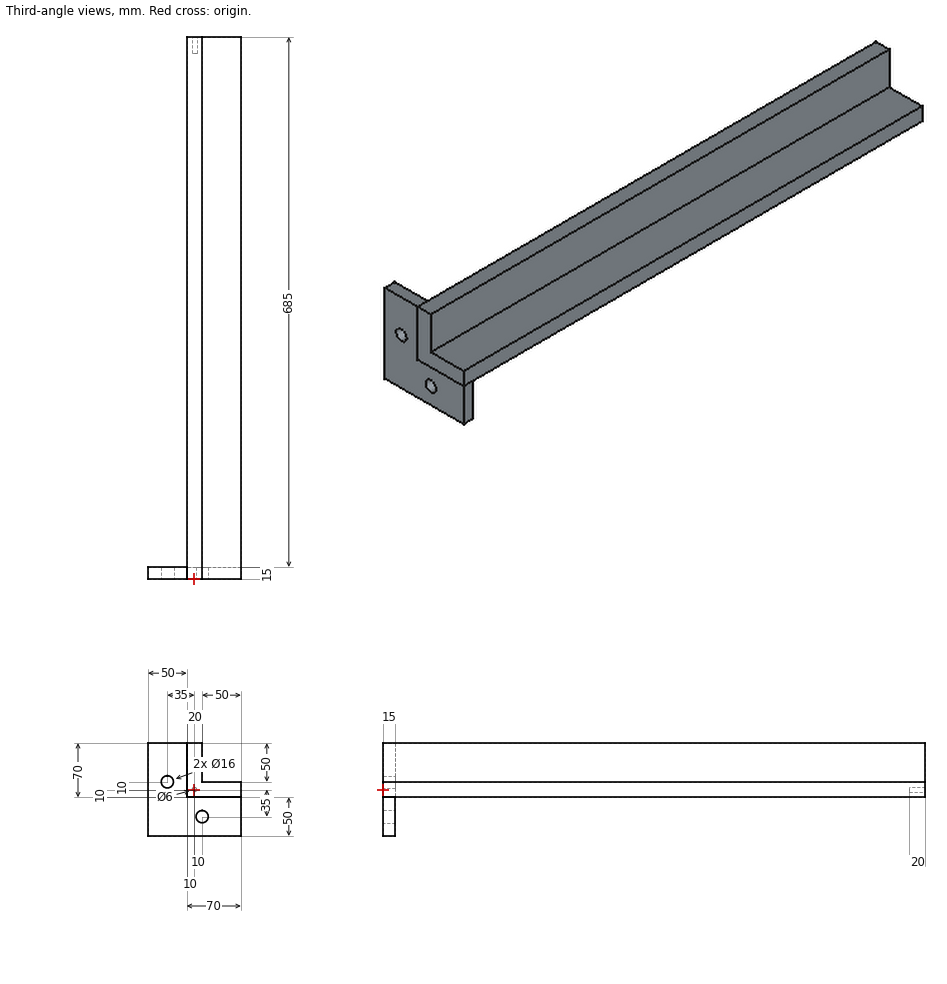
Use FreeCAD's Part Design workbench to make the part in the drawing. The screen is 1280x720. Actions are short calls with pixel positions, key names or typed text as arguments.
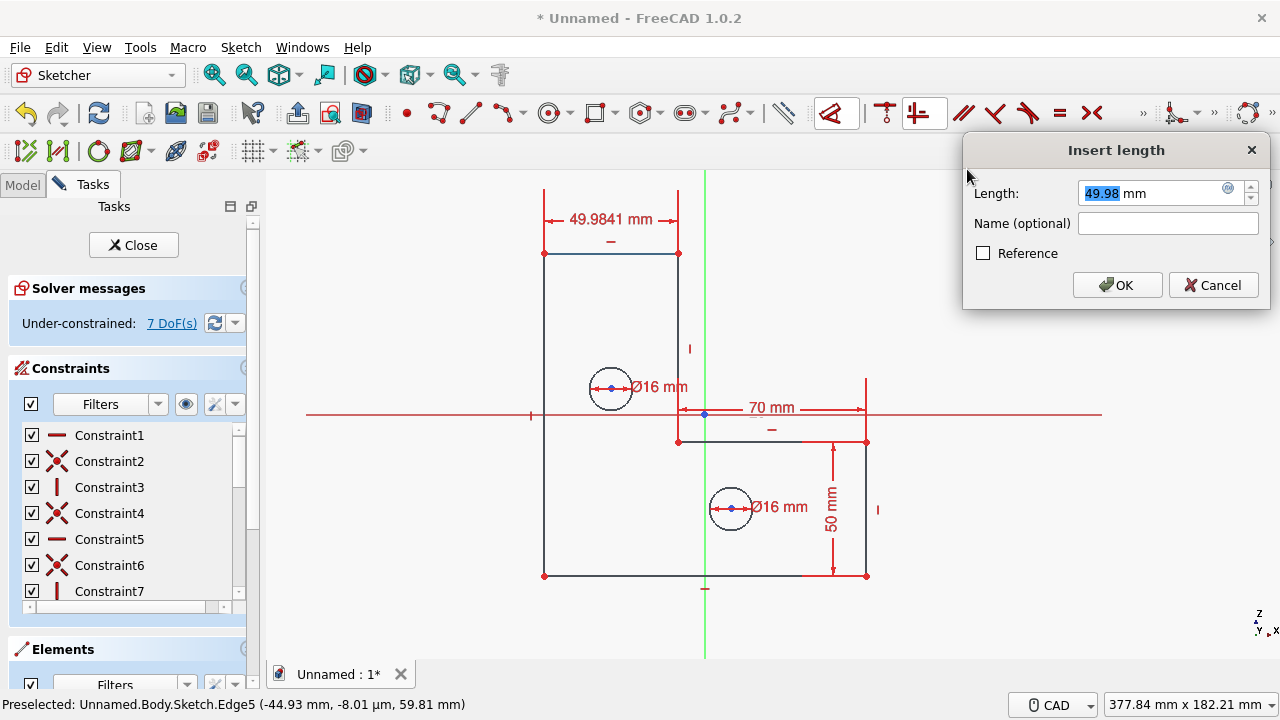
text(50)
key(Return)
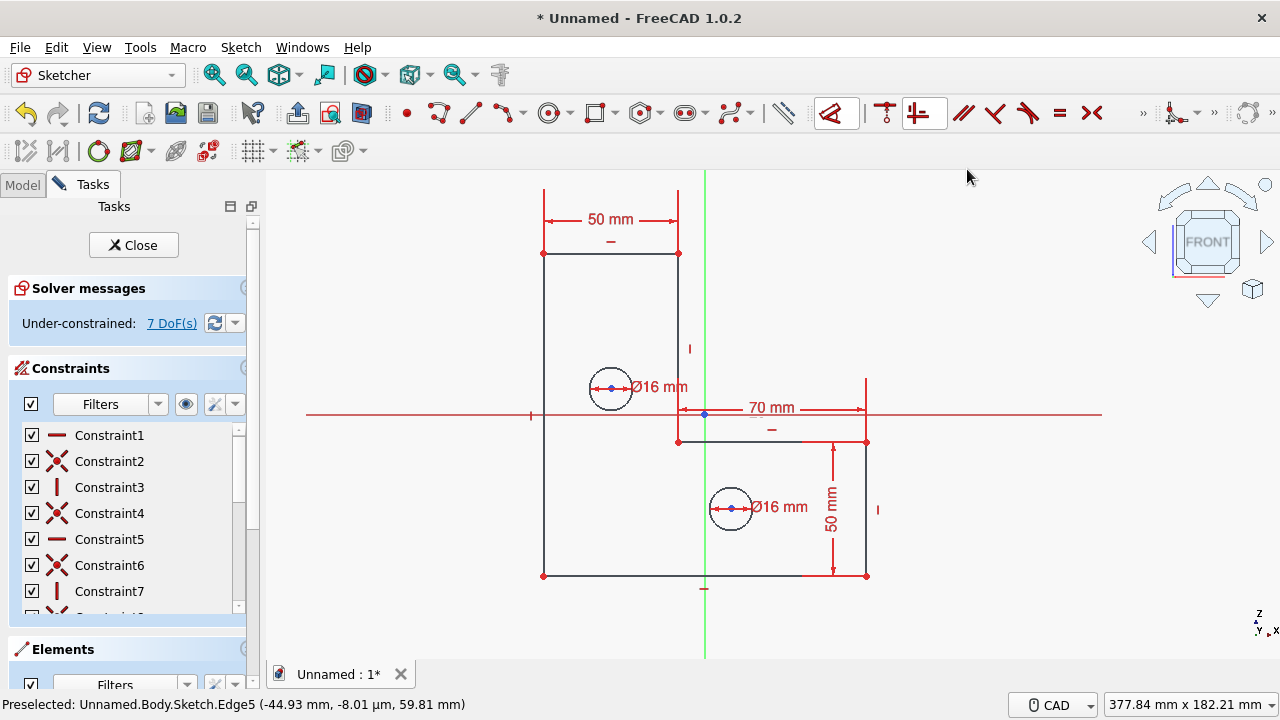
click(678, 310)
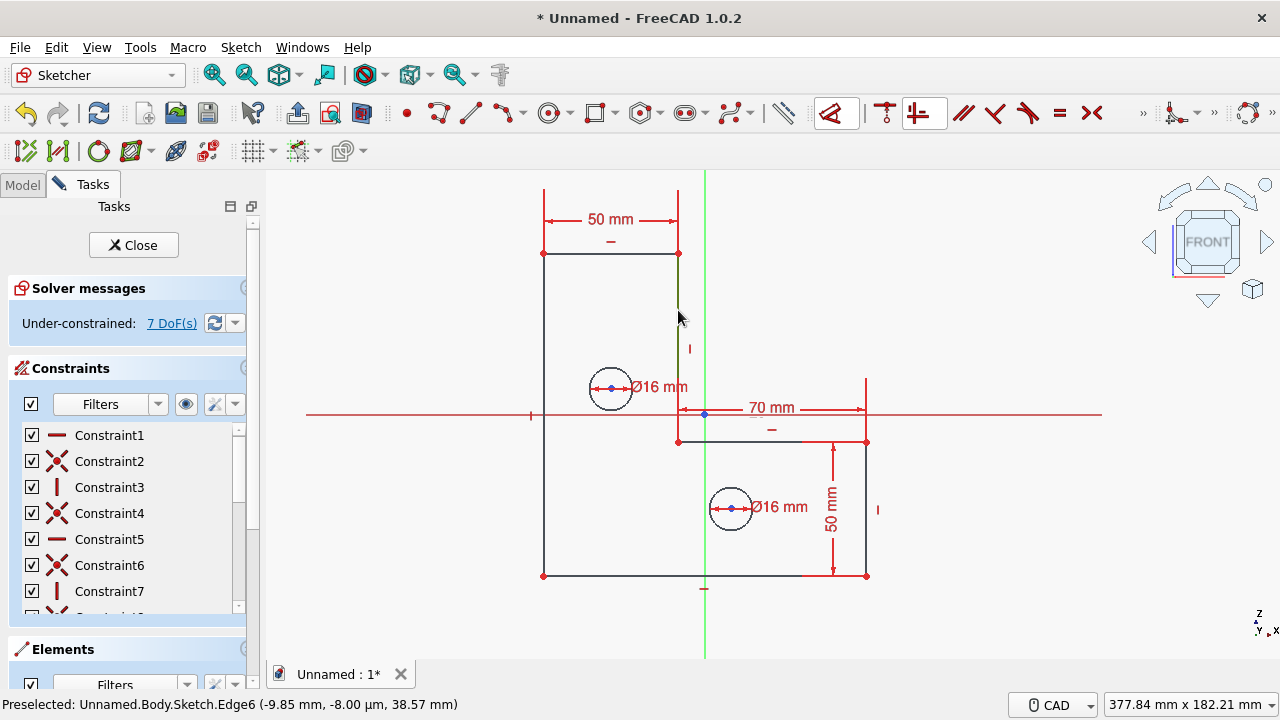
key(i)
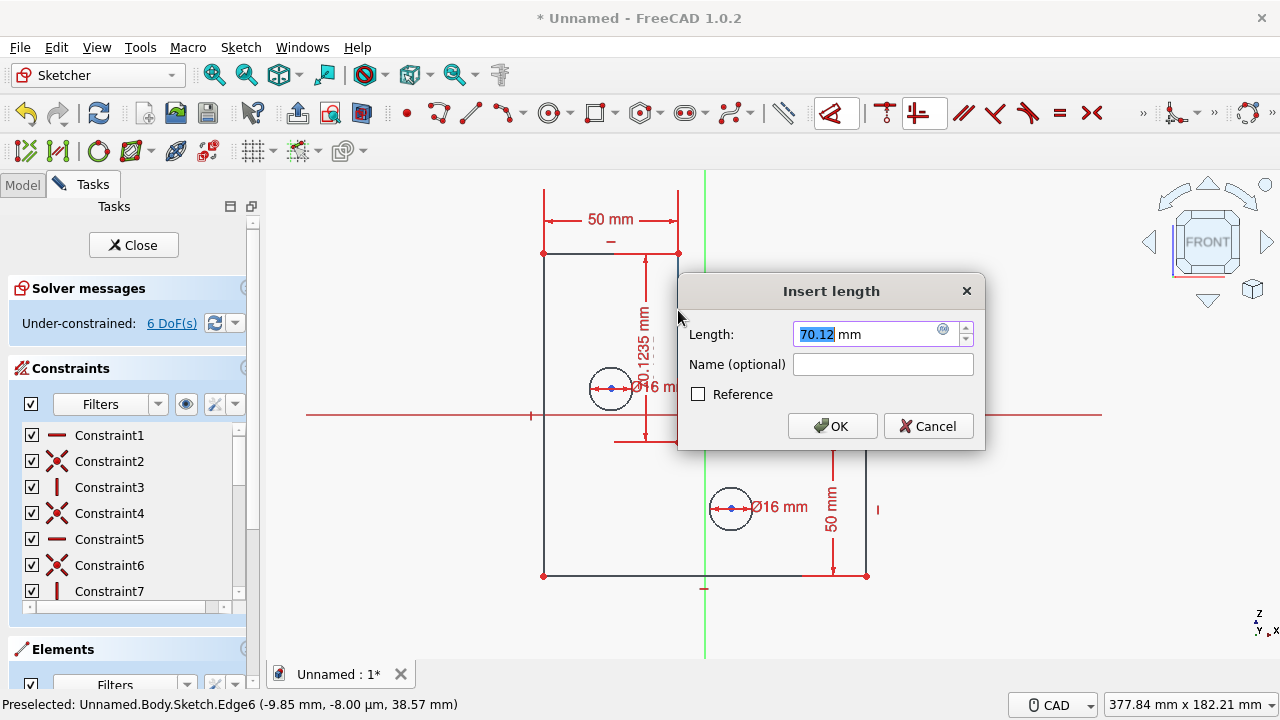
text(70)
key(Return)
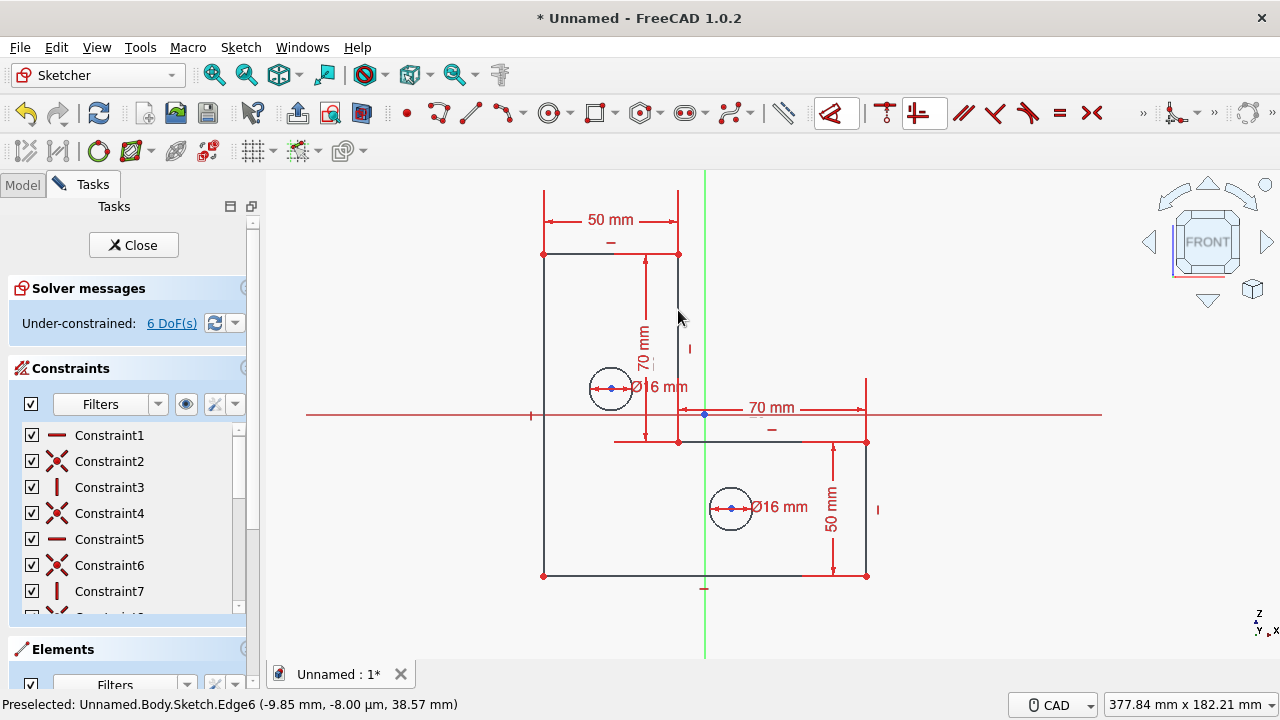
click(611, 389)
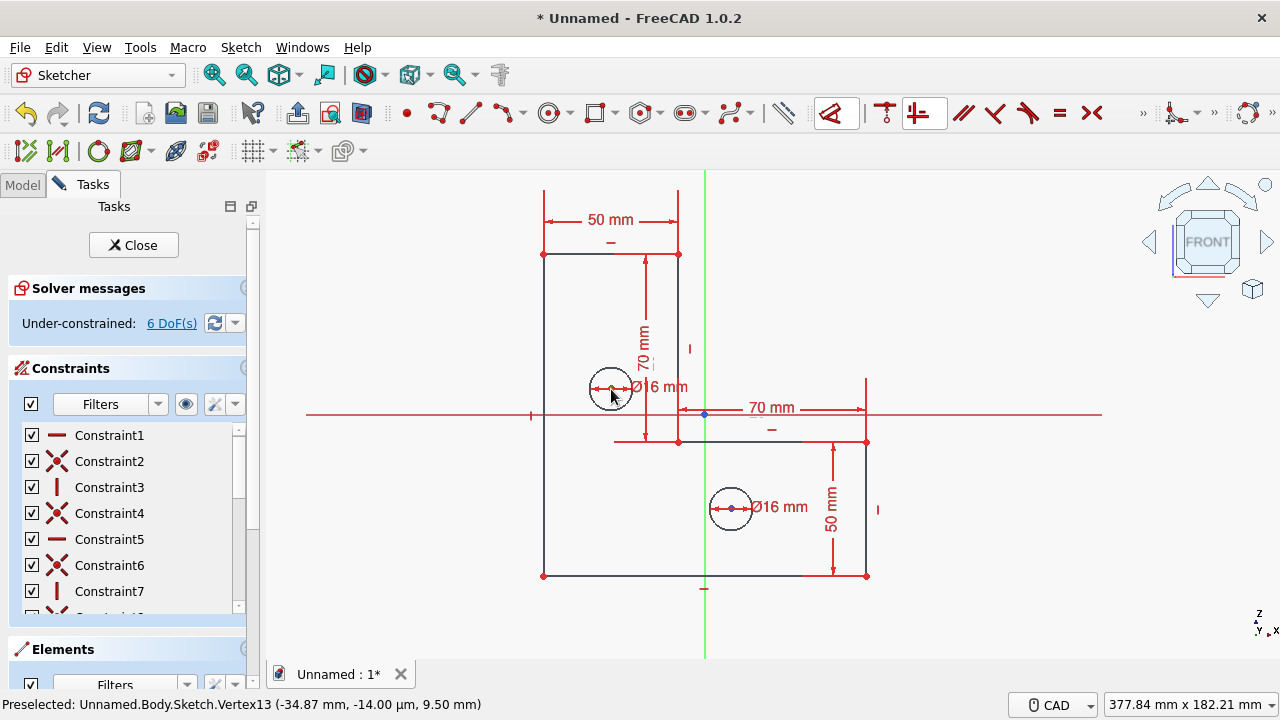
key(l)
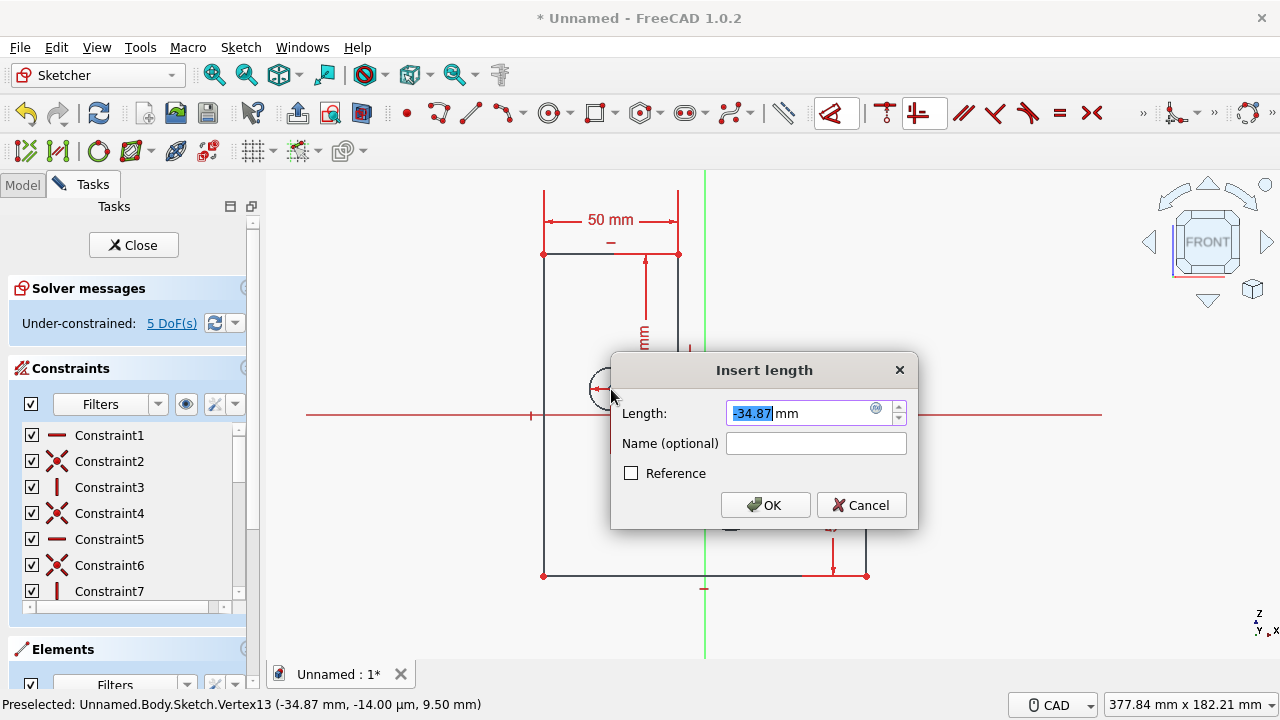
text(-35)
key(Return)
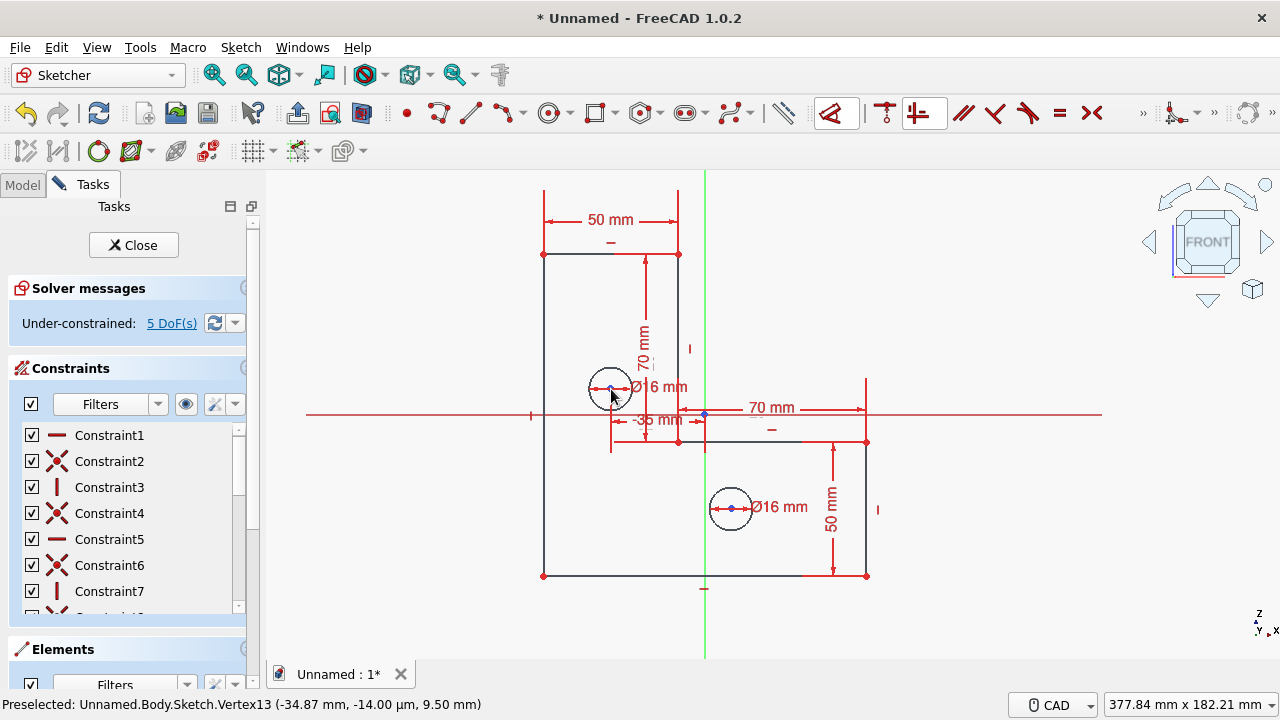
scroll(611, 389, up, 2)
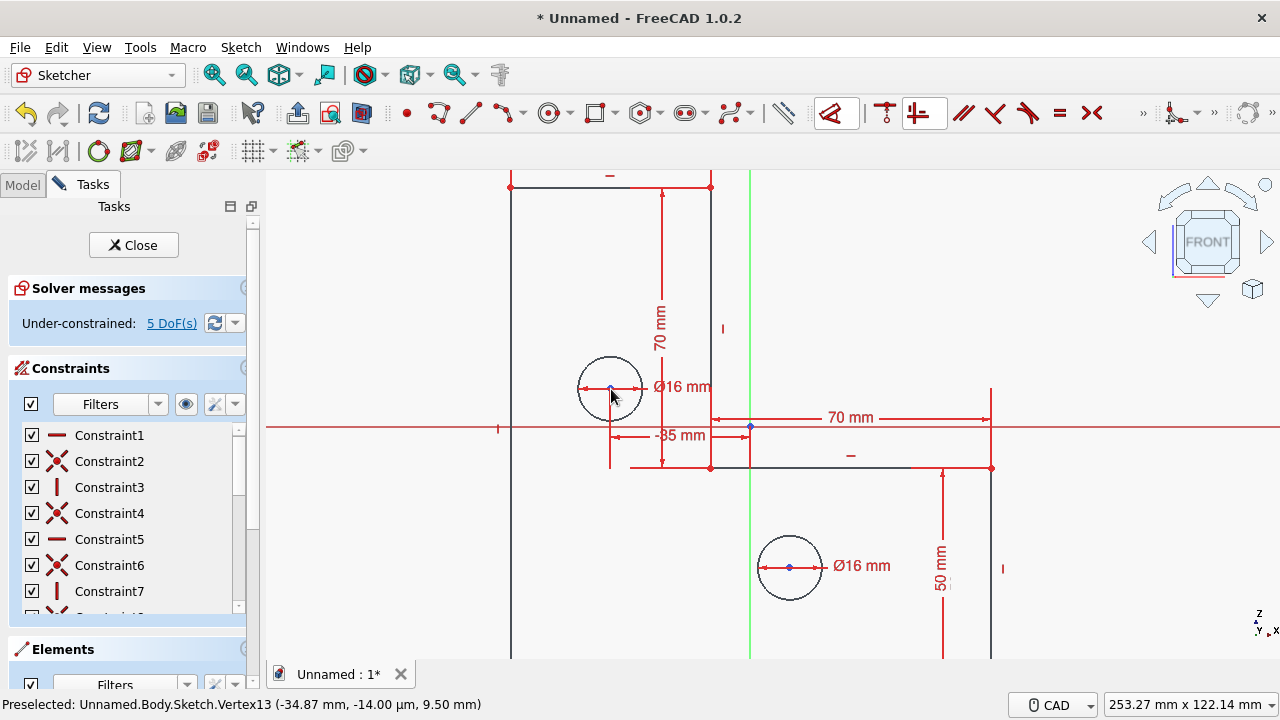
click(610, 389)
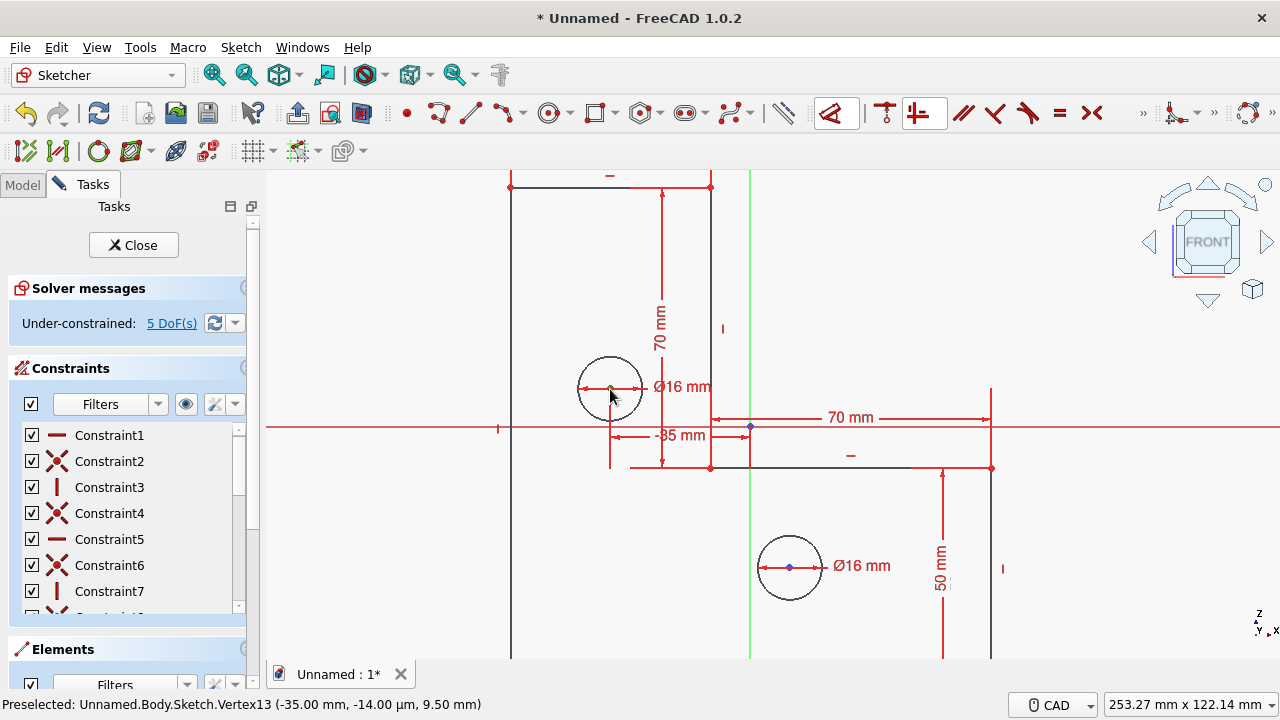
key(i)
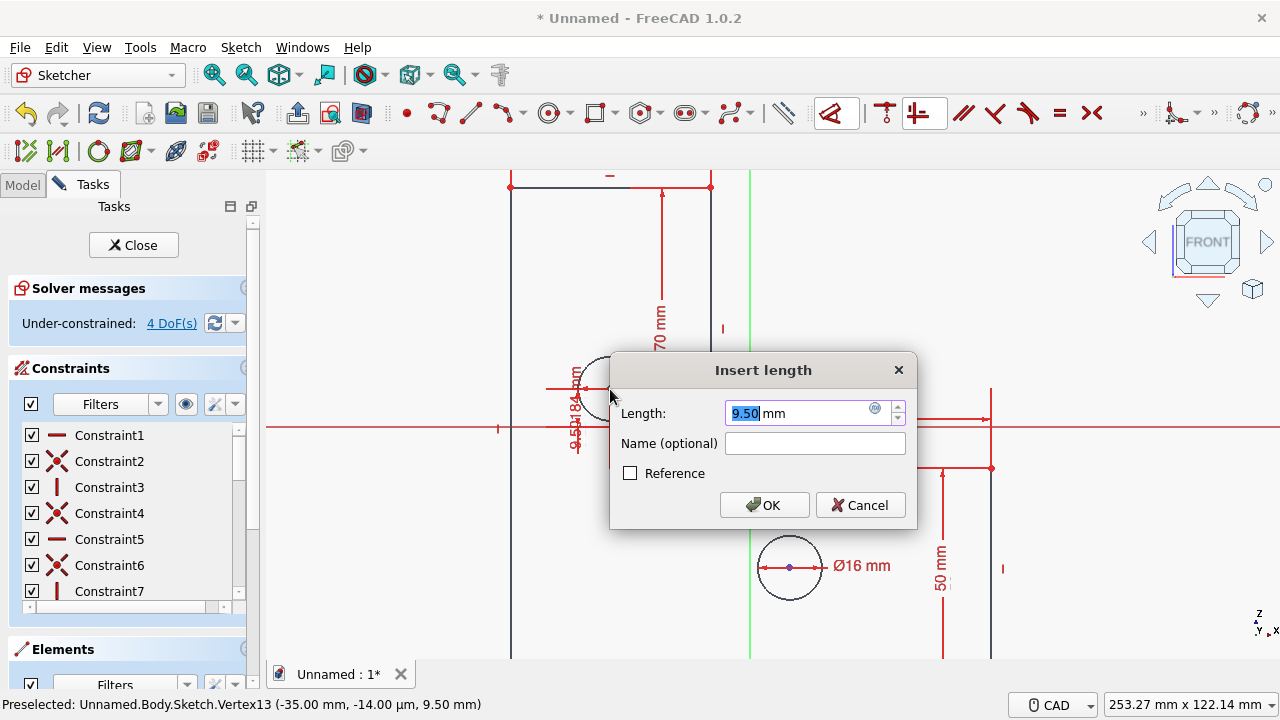
text(10)
key(Return)